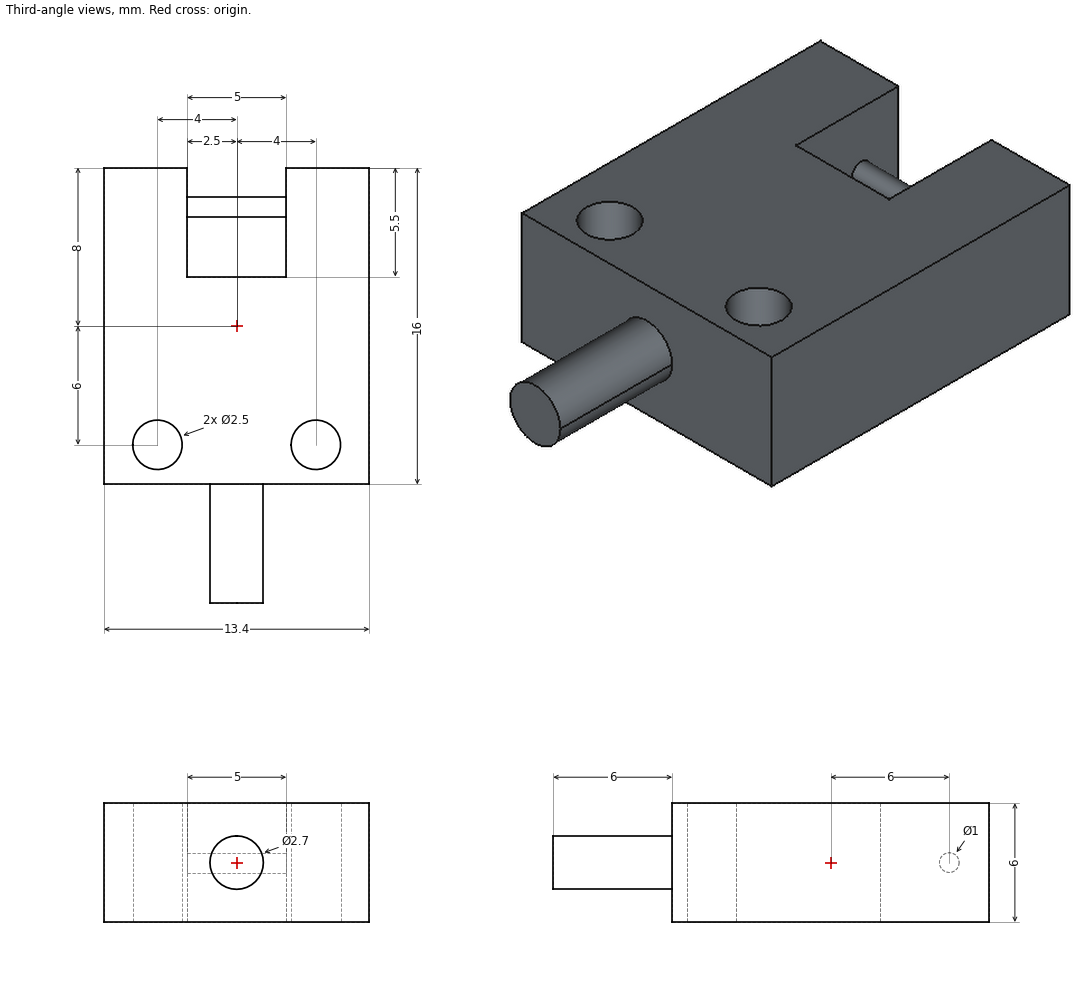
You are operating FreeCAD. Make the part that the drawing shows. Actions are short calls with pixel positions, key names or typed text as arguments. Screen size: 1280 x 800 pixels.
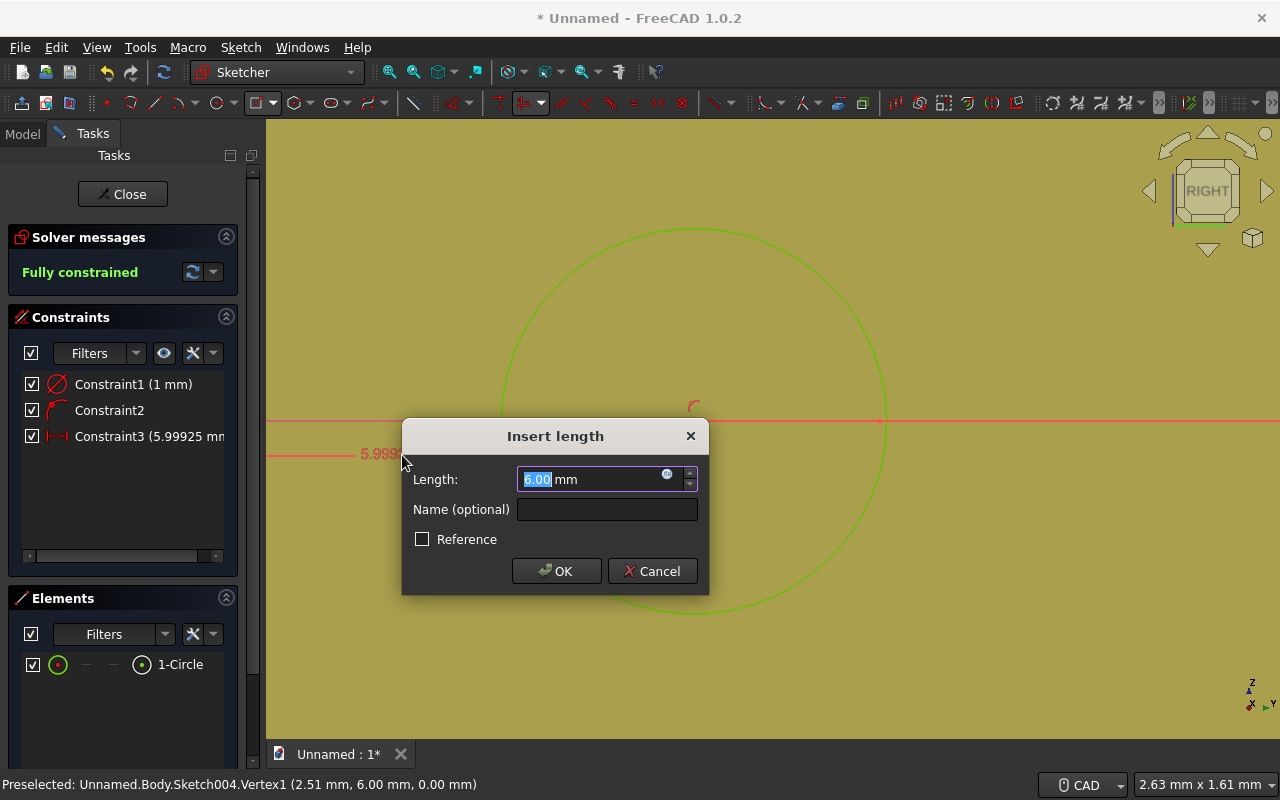
text(6)
key(Return)
key(Escape)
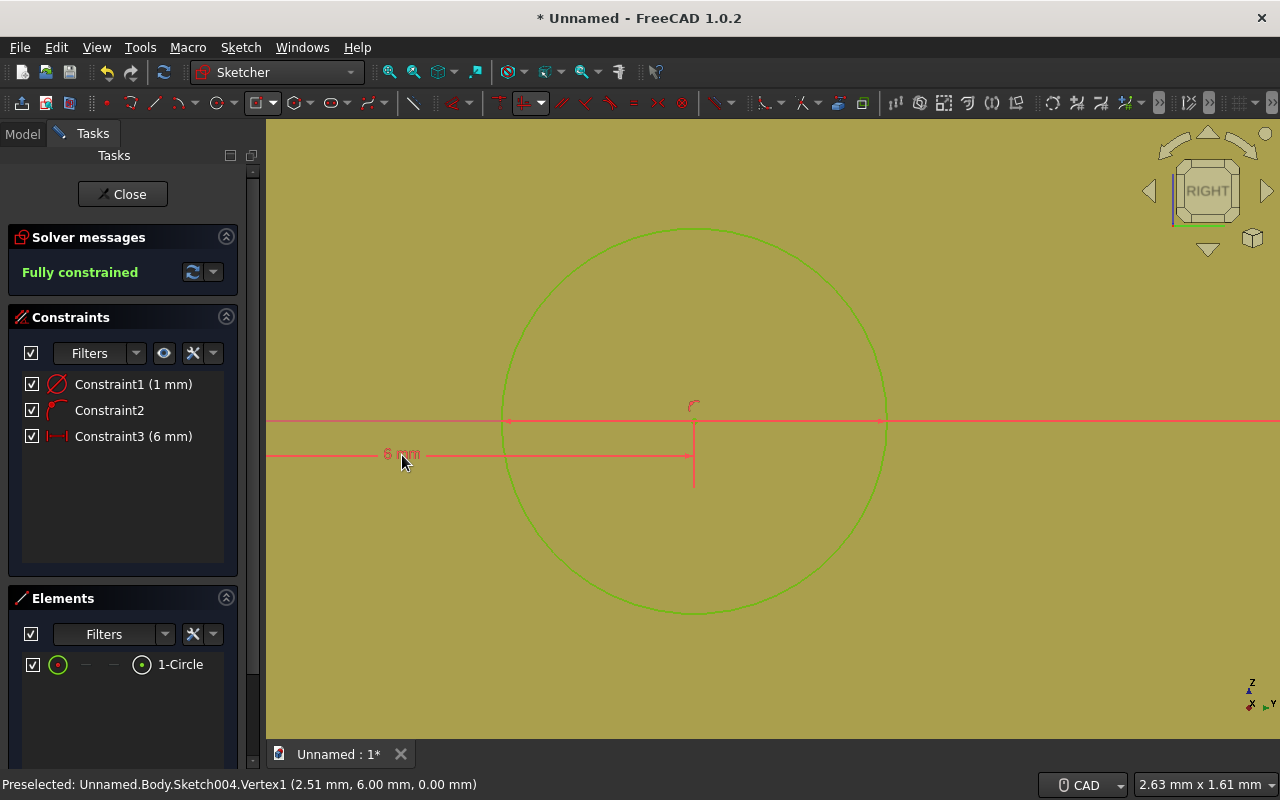
click(123, 194)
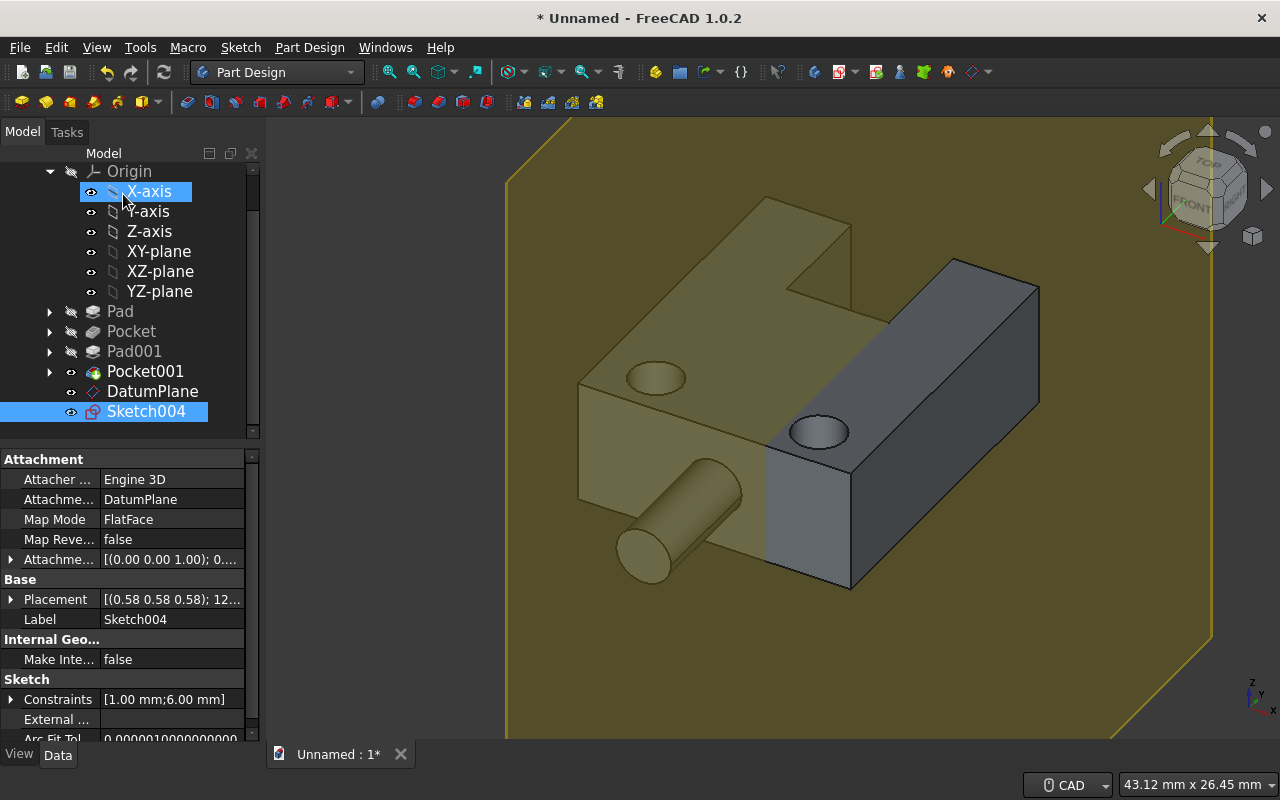
click(22, 102)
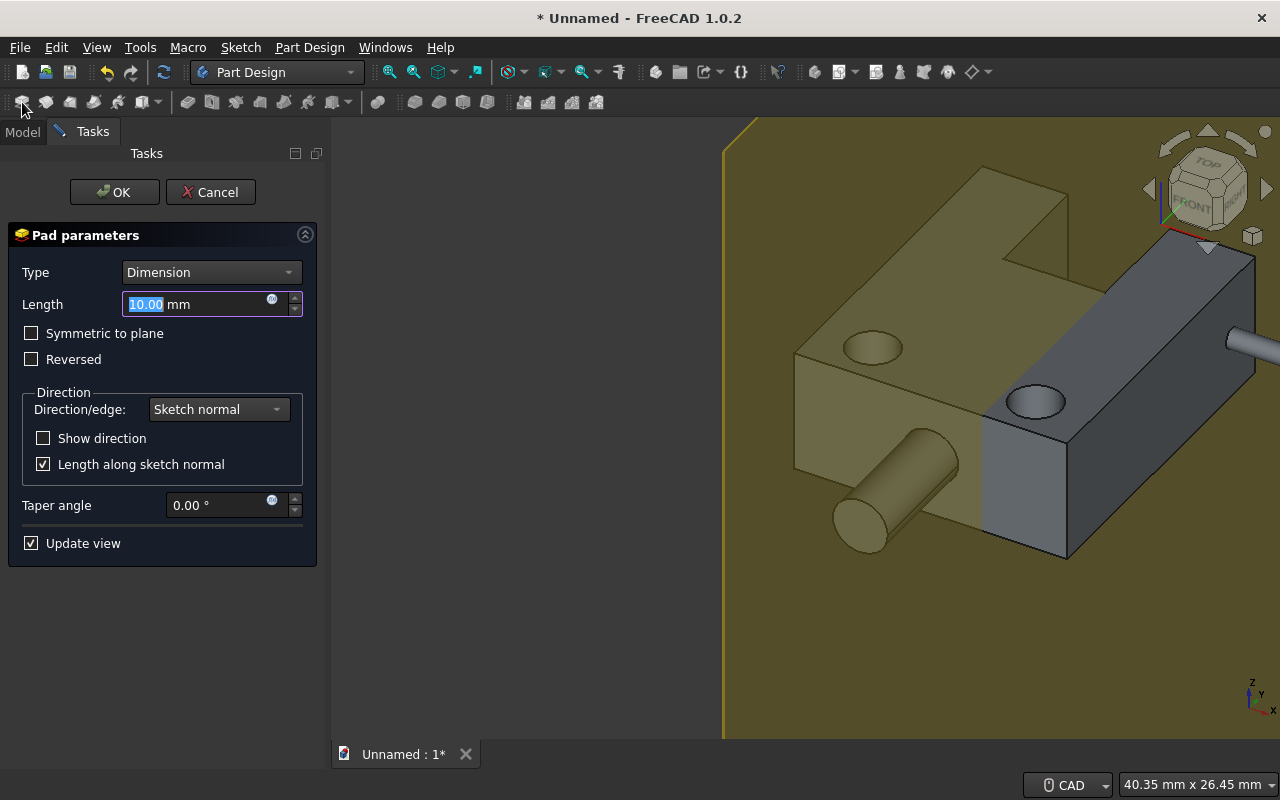
text(5)
key(Tab)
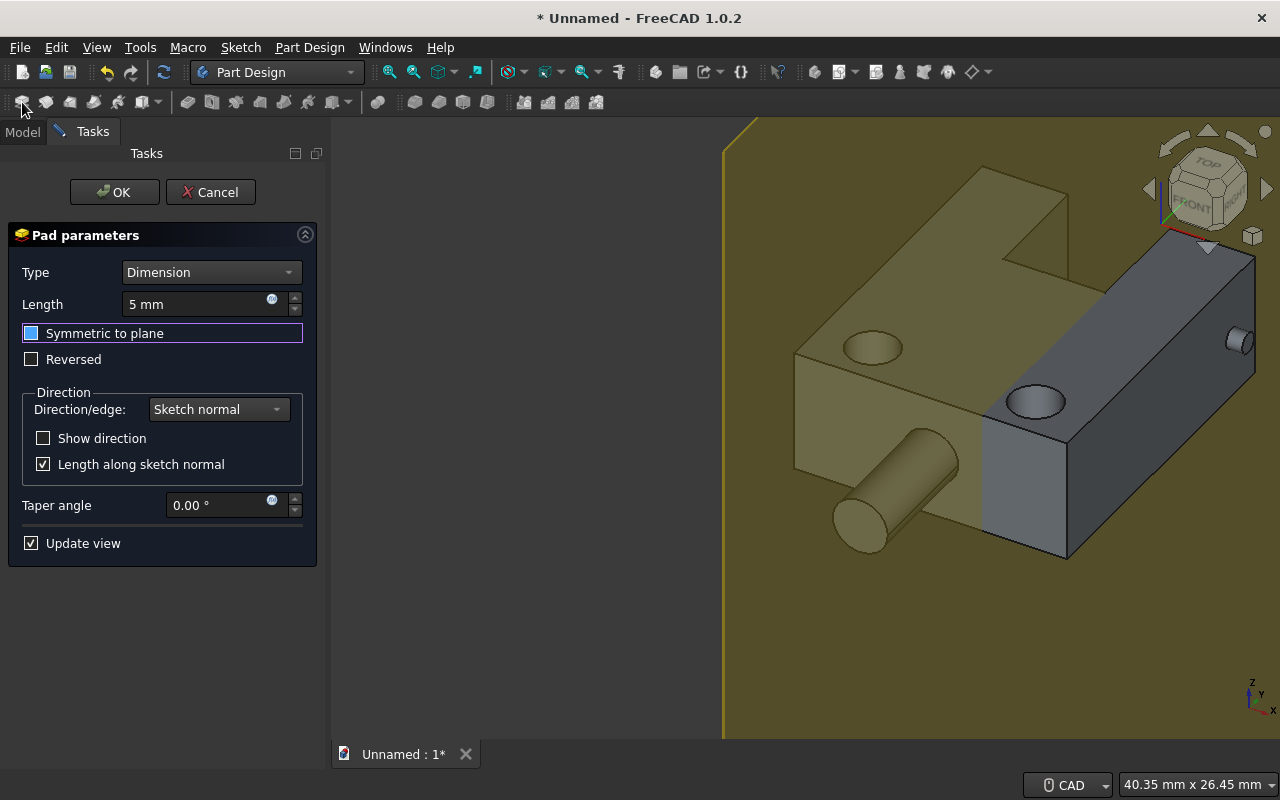
click(30, 359)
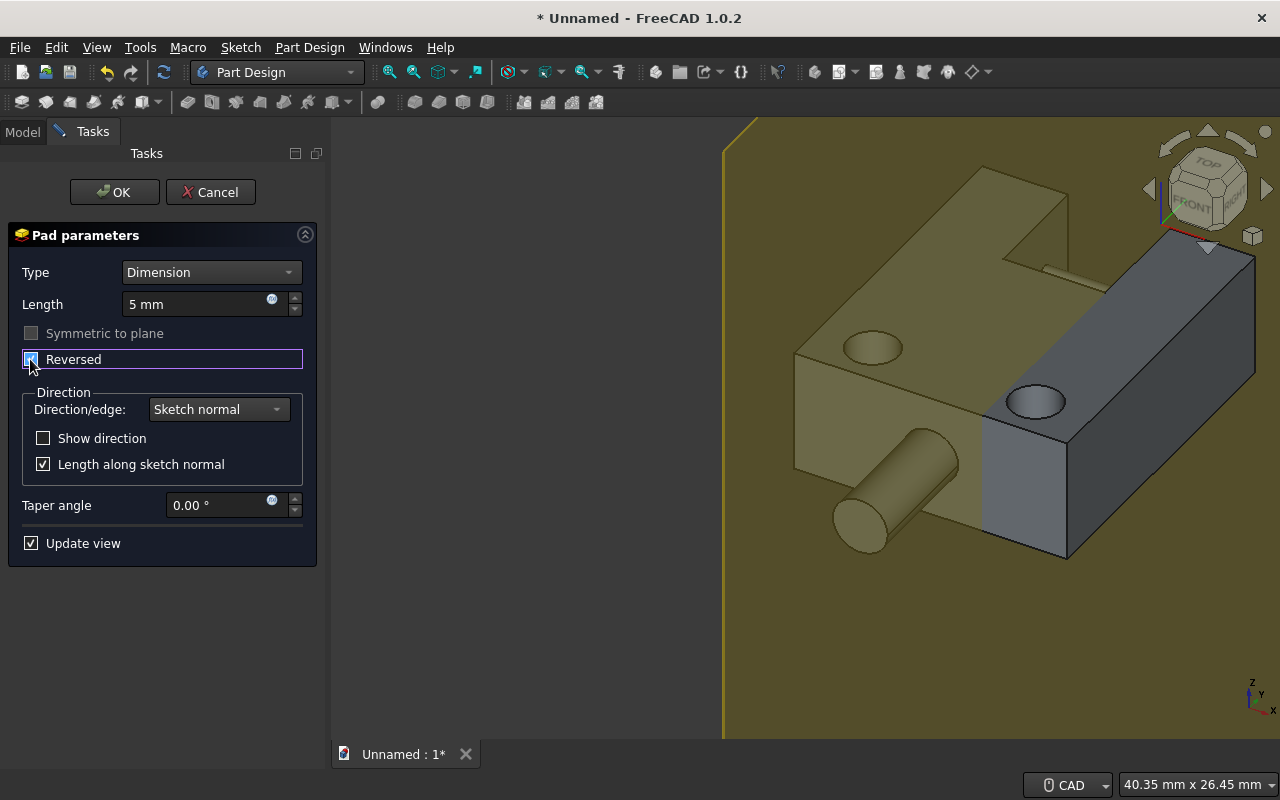
click(115, 192)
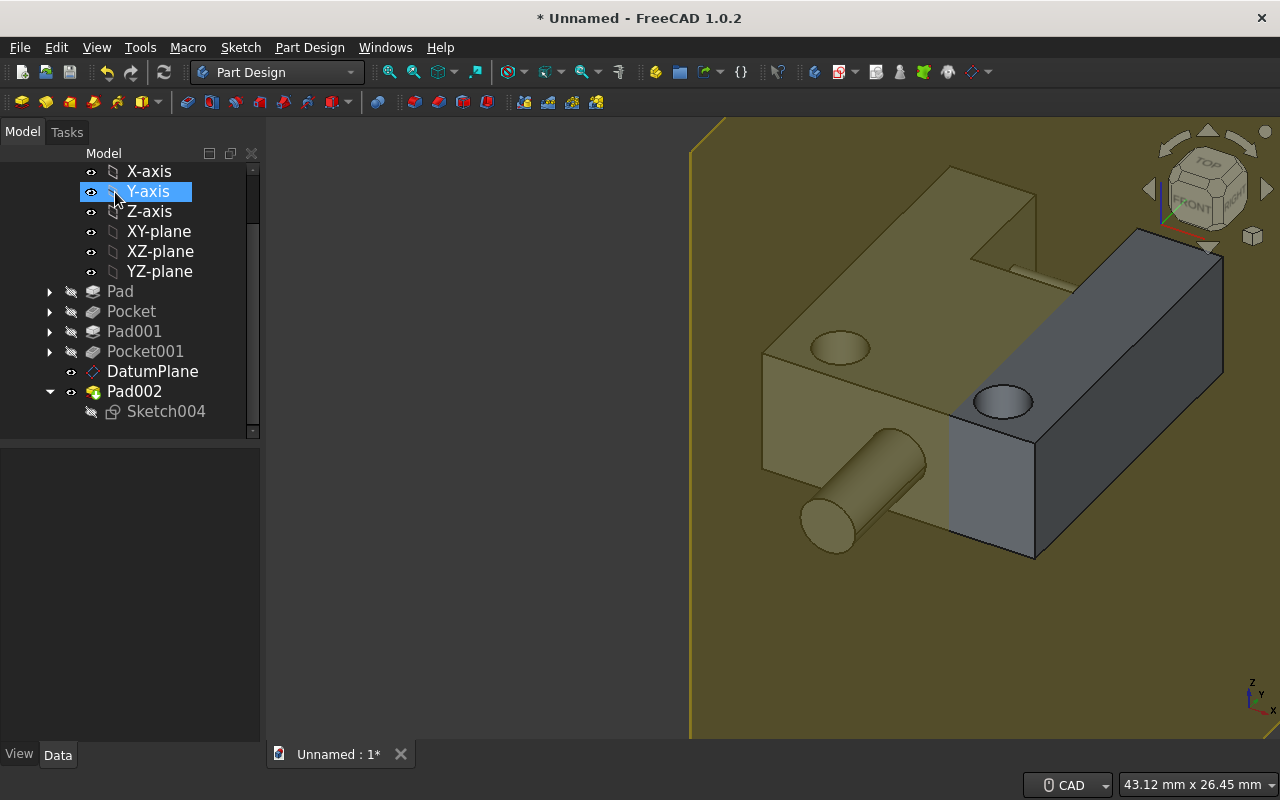
click(116, 372)
key(space)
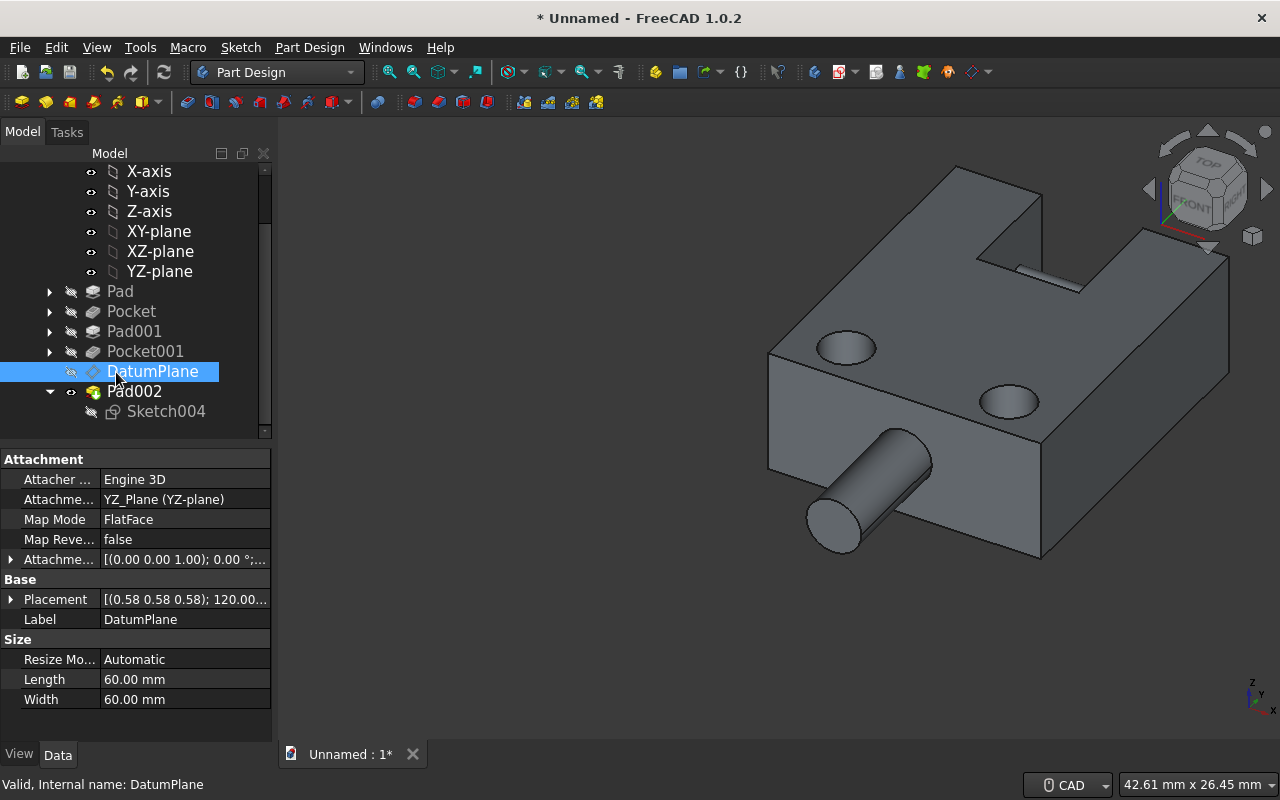
key(0)